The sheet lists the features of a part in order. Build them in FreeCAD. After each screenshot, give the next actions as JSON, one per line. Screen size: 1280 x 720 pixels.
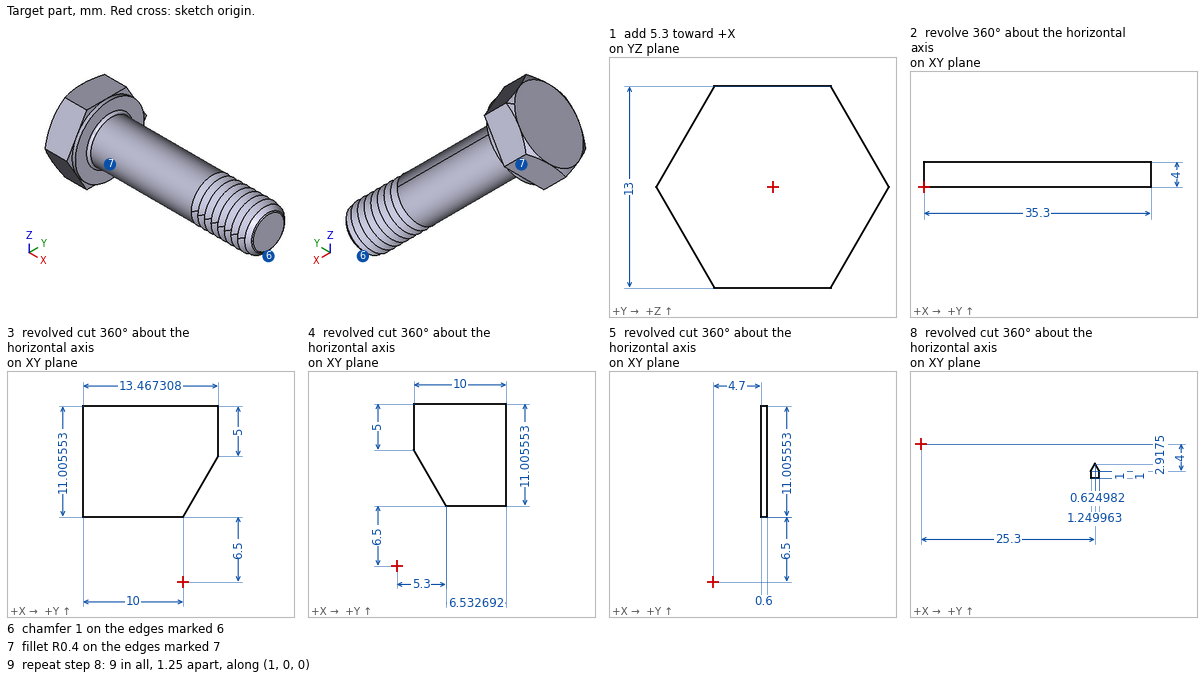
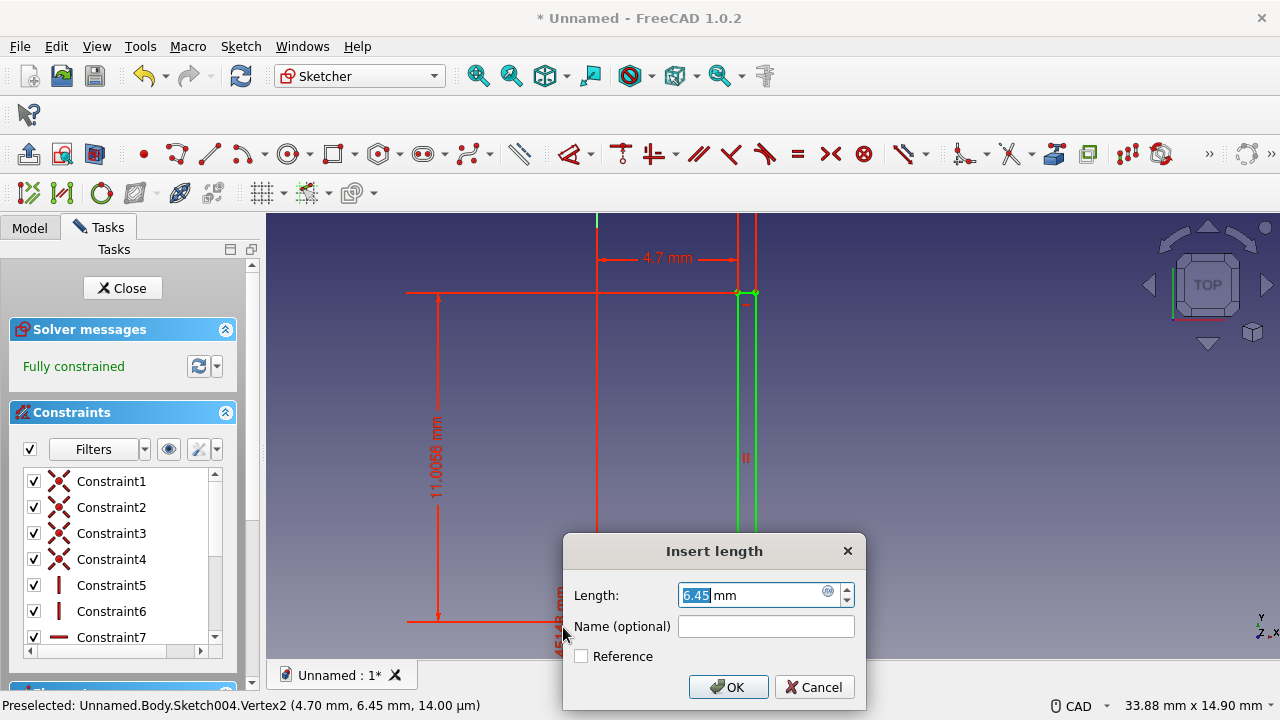
{"action": "type", "text": "6.5"}
{"action": "key", "text": "Return"}
{"action": "key", "text": "Escape"}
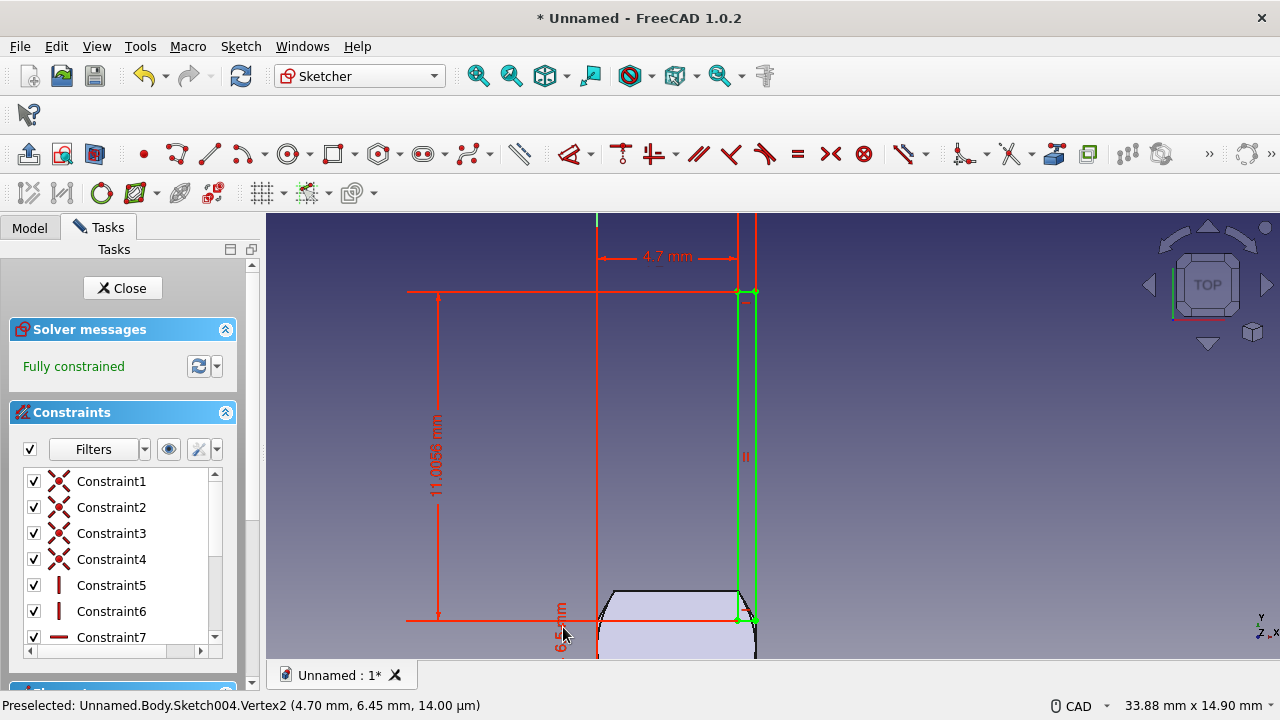
{"action": "left_click", "coordinate": [123, 288]}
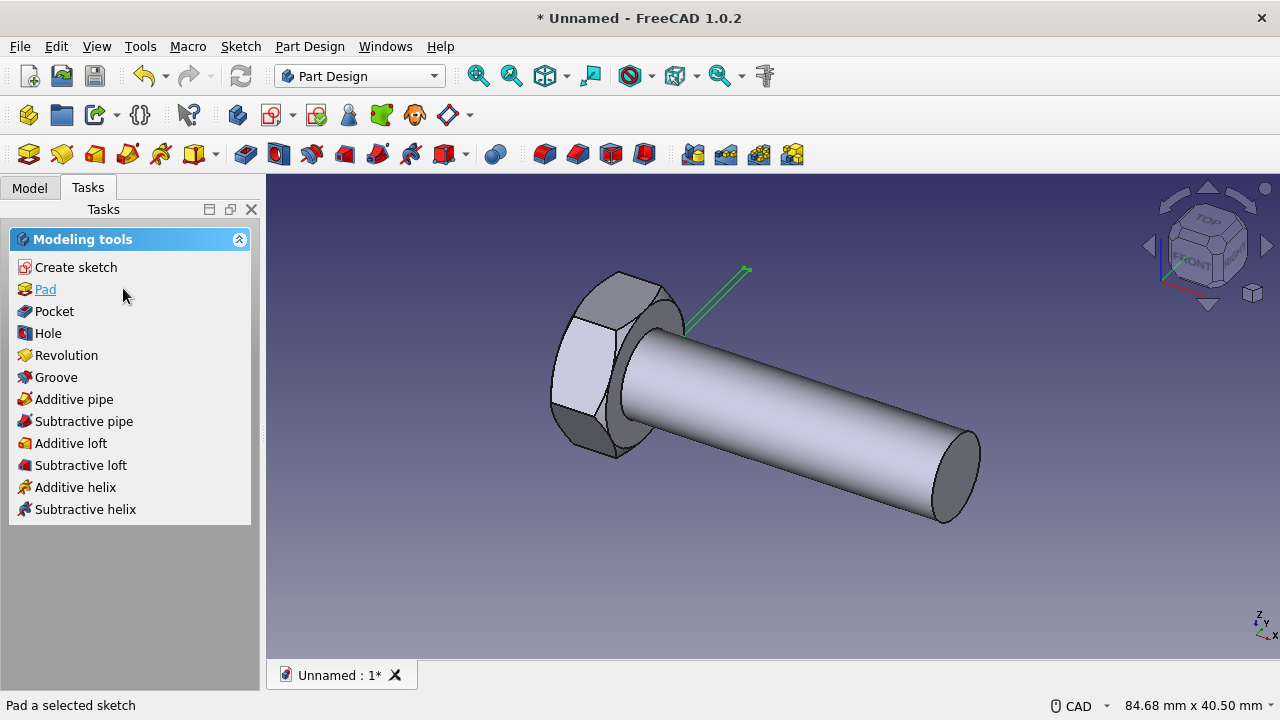
{"action": "left_click", "coordinate": [312, 154]}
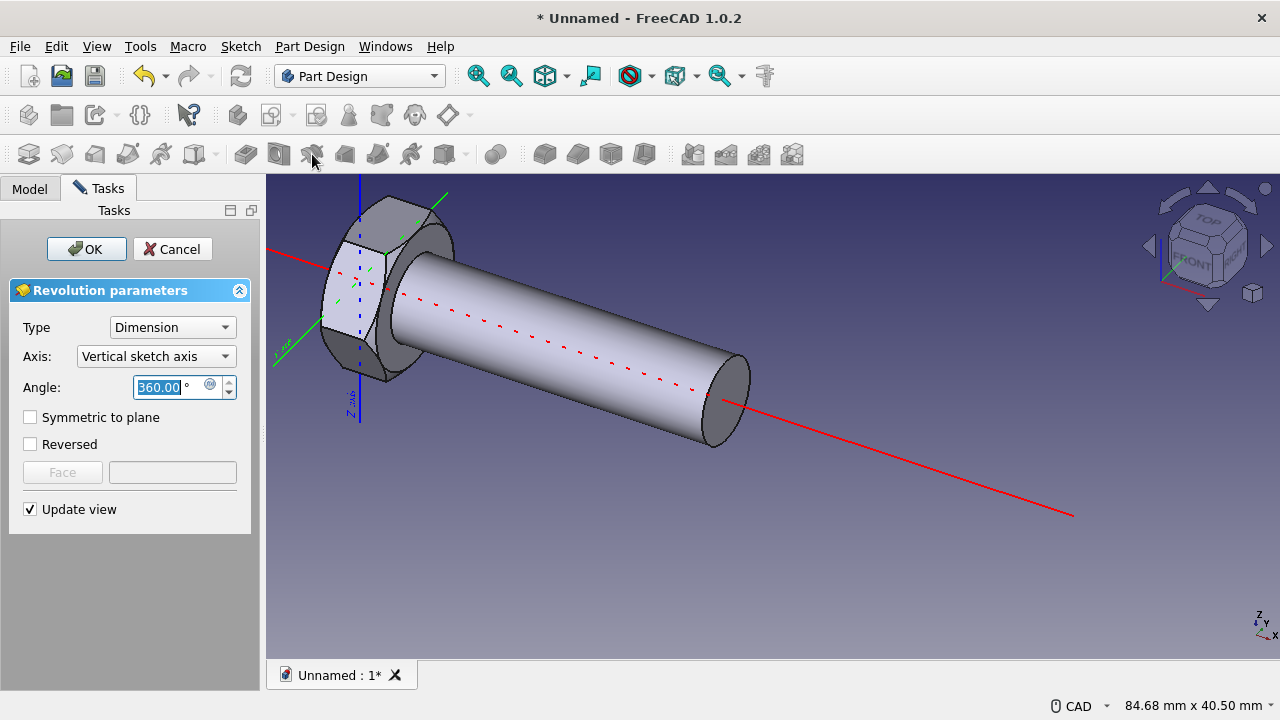
{"action": "left_click", "coordinate": [157, 356]}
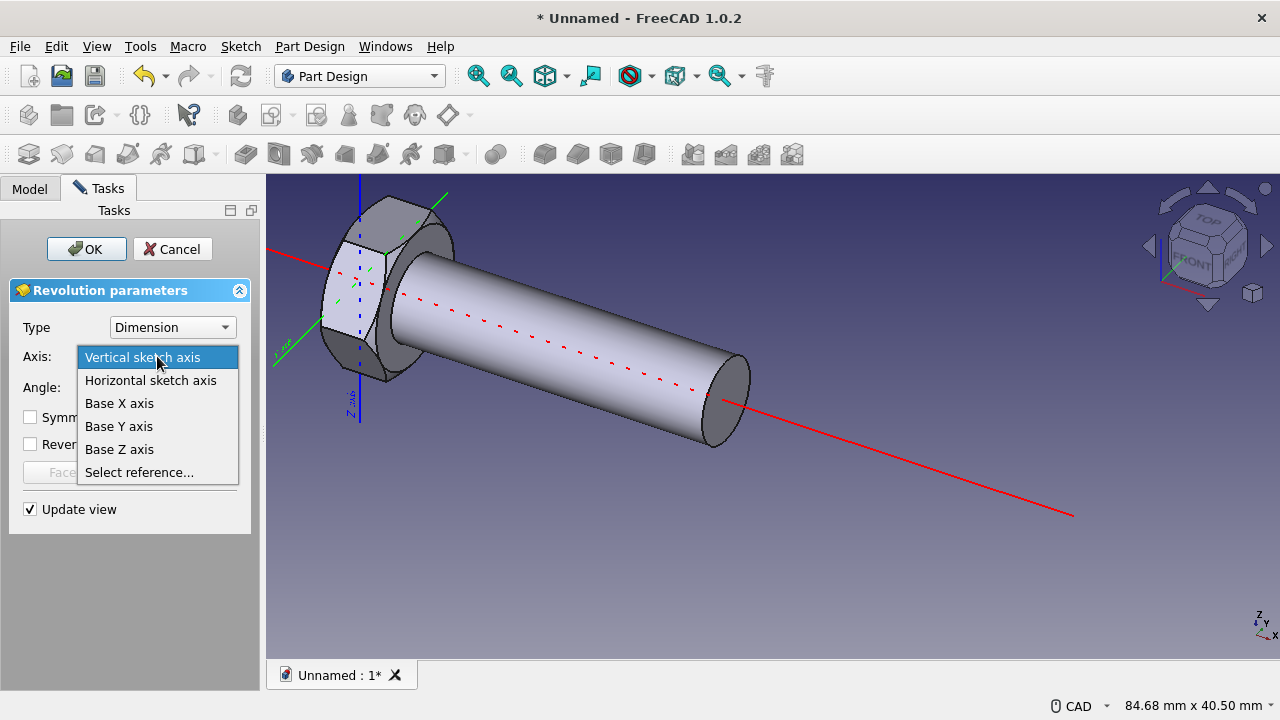
{"action": "left_click", "coordinate": [156, 380]}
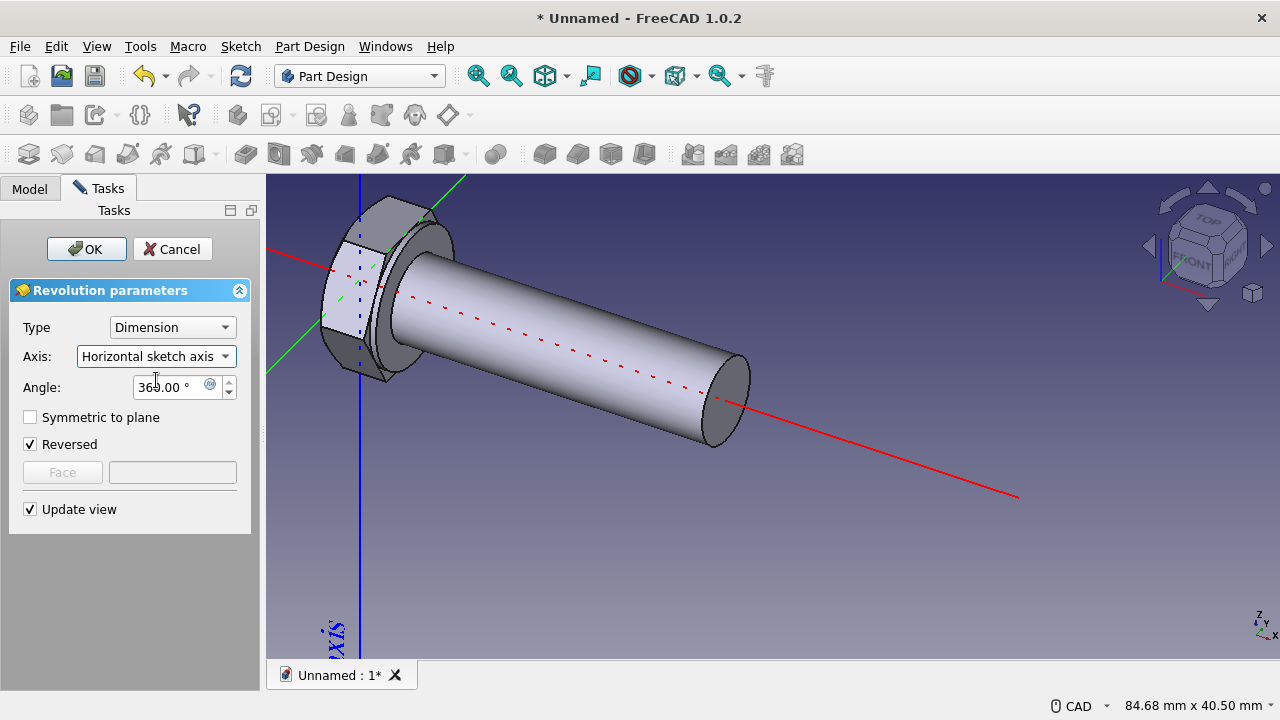
{"action": "left_click", "coordinate": [87, 249]}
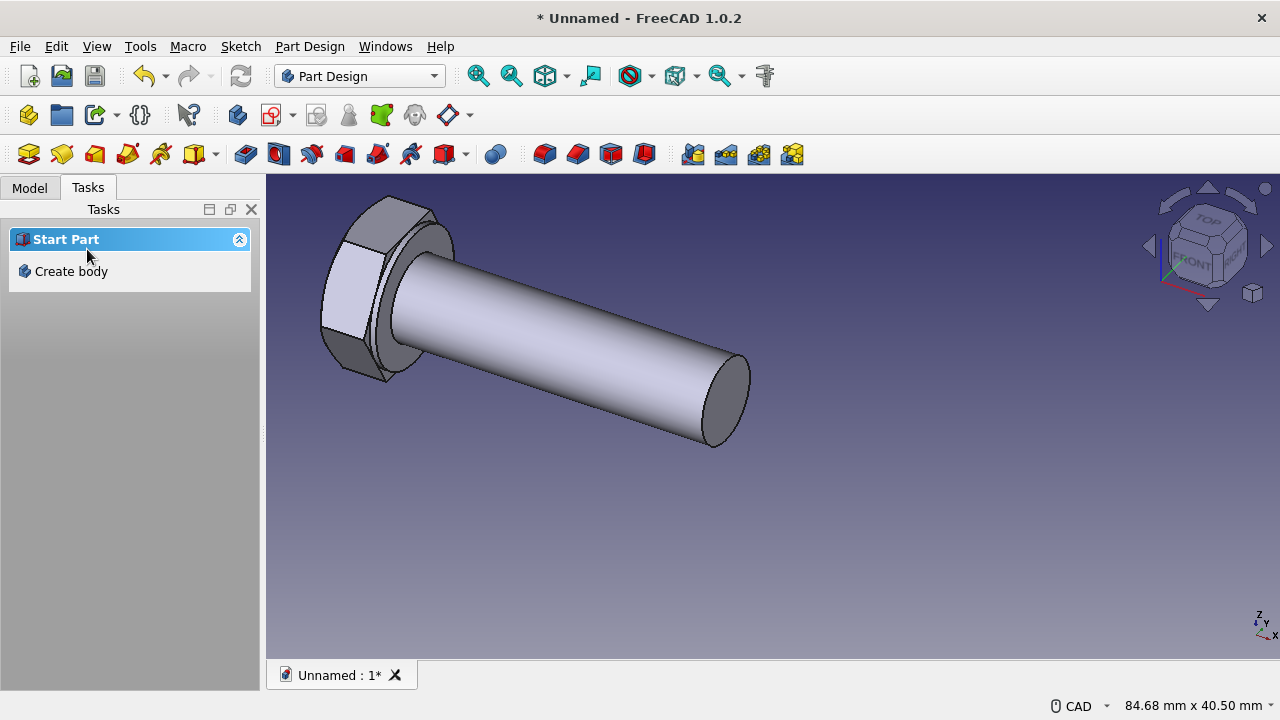
{"action": "left_click", "coordinate": [479, 76]}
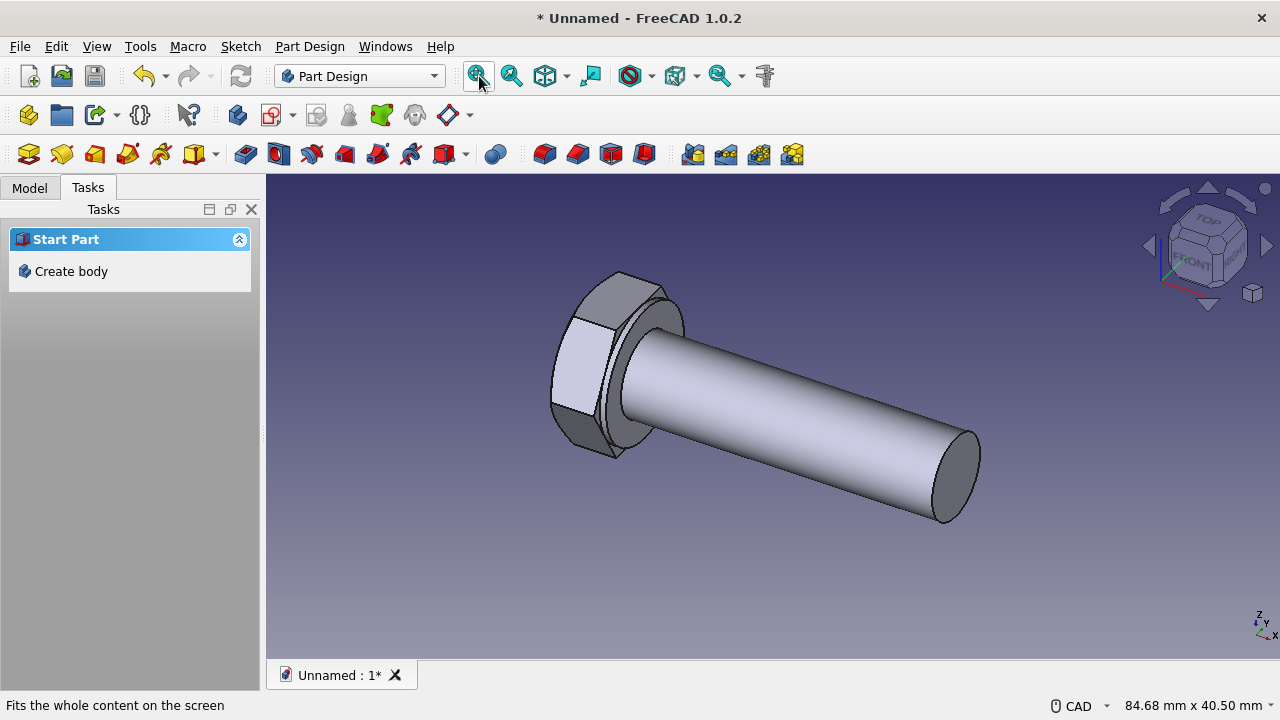
{"action": "left_click", "coordinate": [932, 500]}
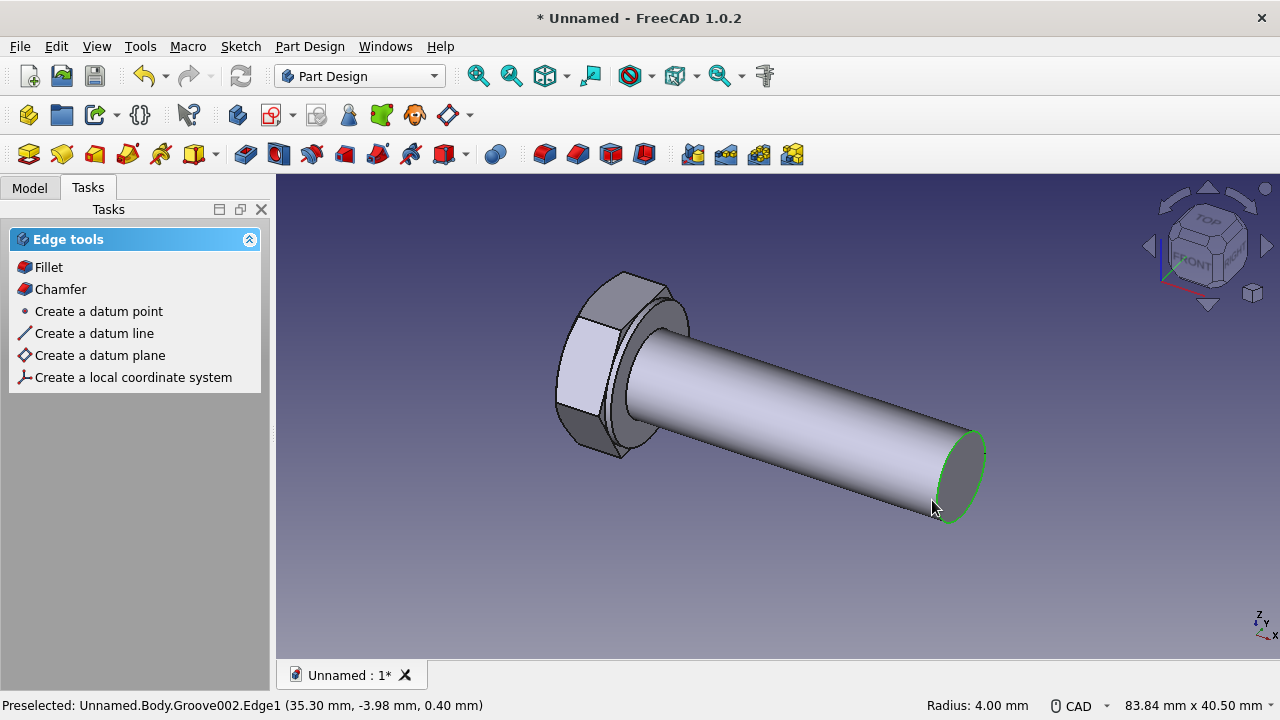
{"action": "left_click", "coordinate": [578, 154]}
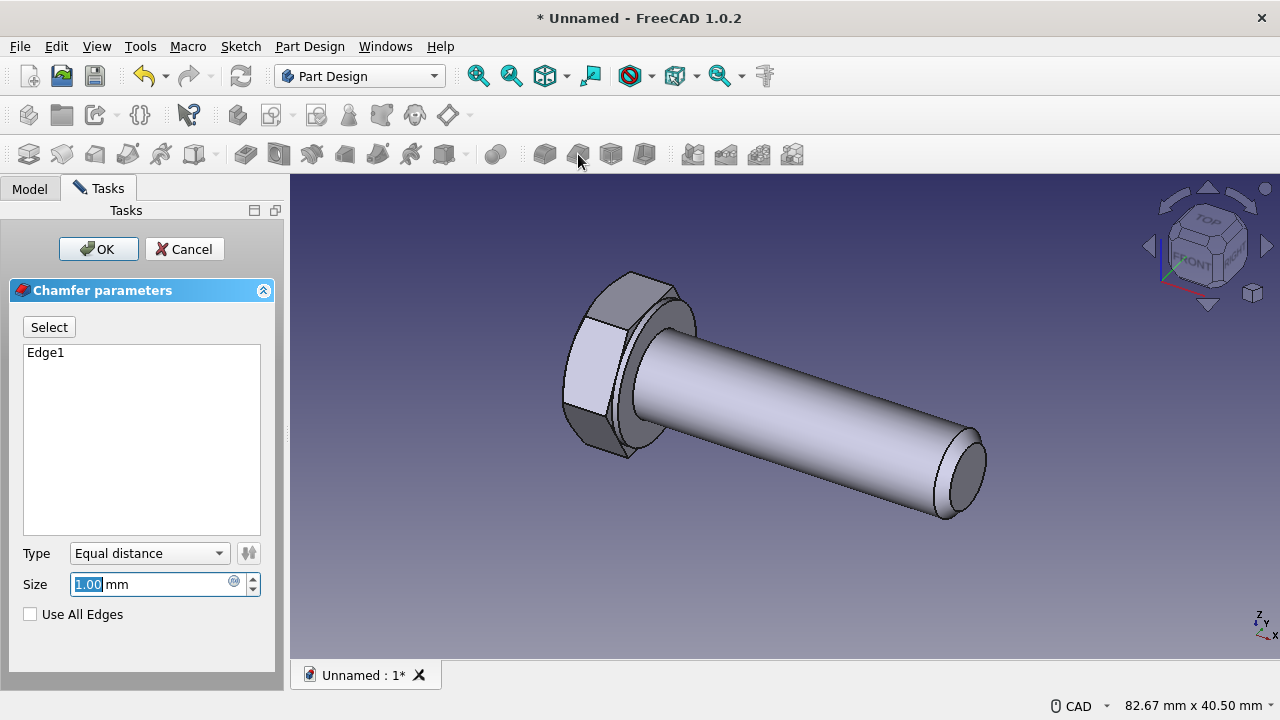
{"action": "type", "text": "1"}
{"action": "key", "text": "Tab"}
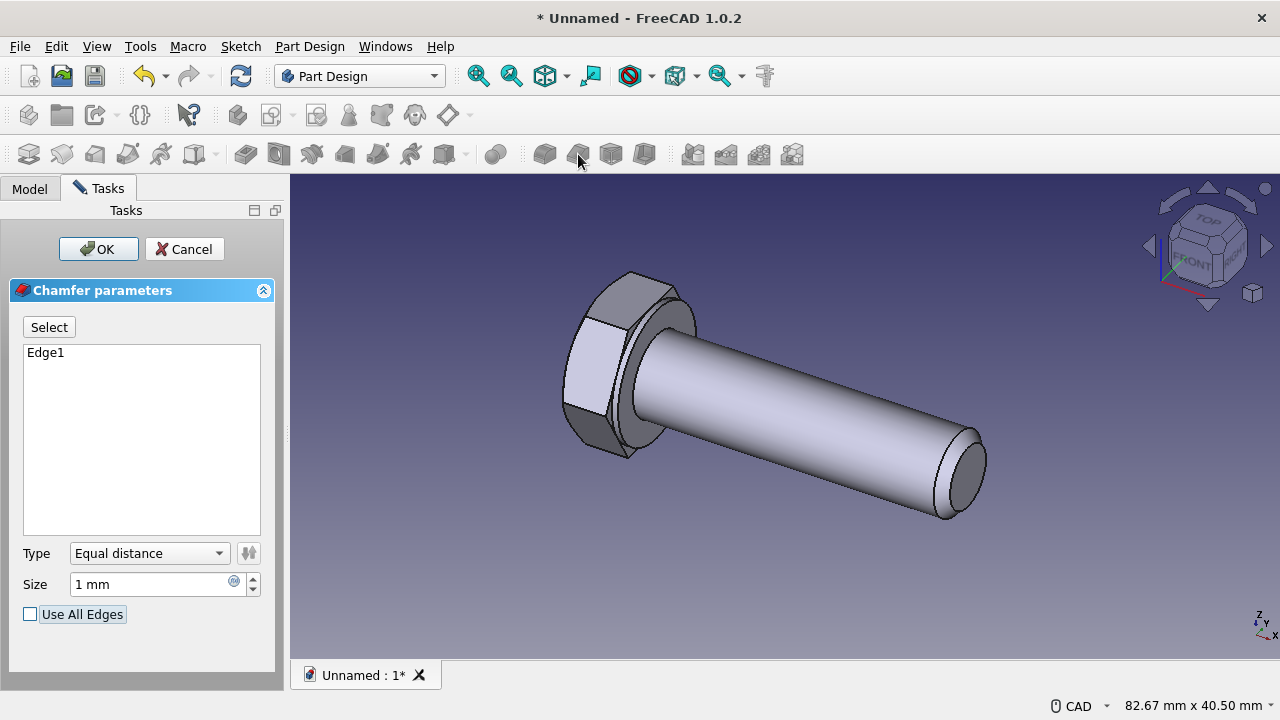
{"action": "left_click", "coordinate": [99, 249]}